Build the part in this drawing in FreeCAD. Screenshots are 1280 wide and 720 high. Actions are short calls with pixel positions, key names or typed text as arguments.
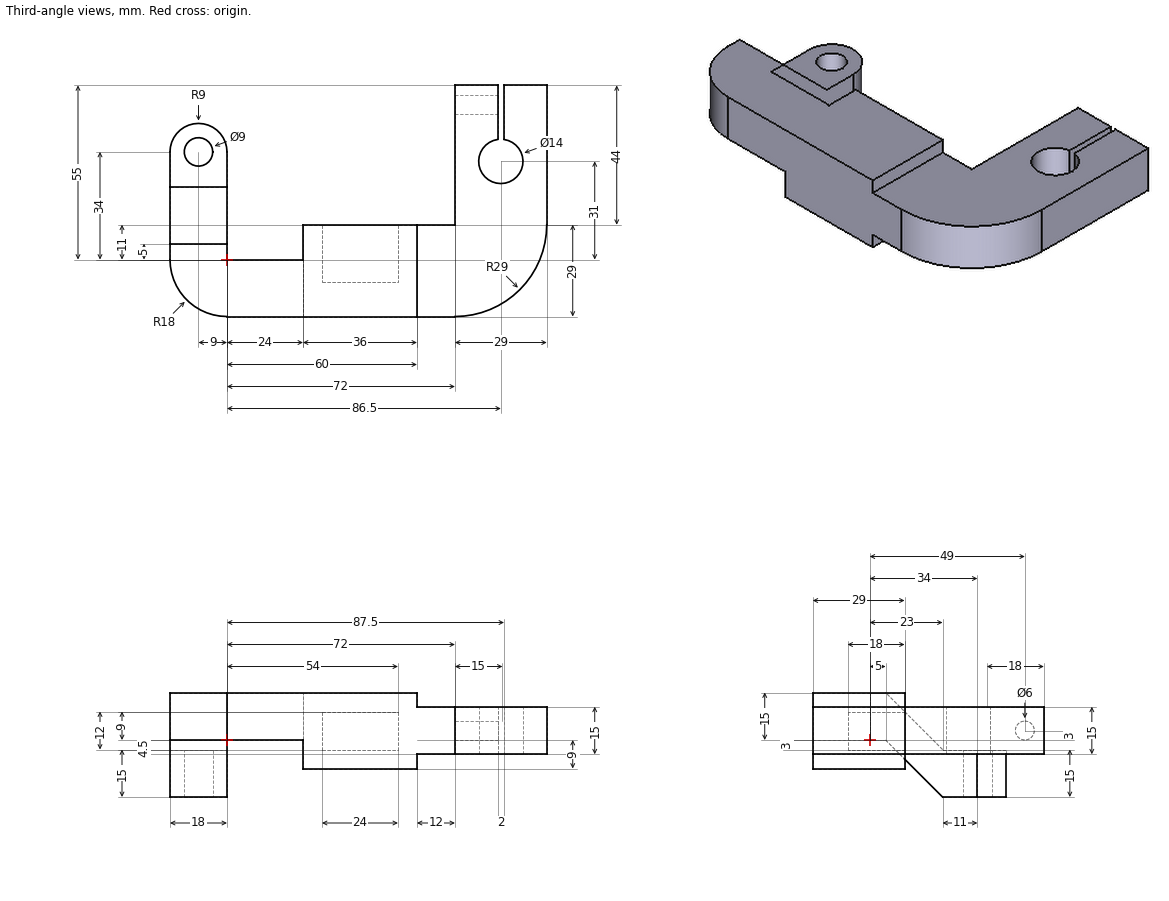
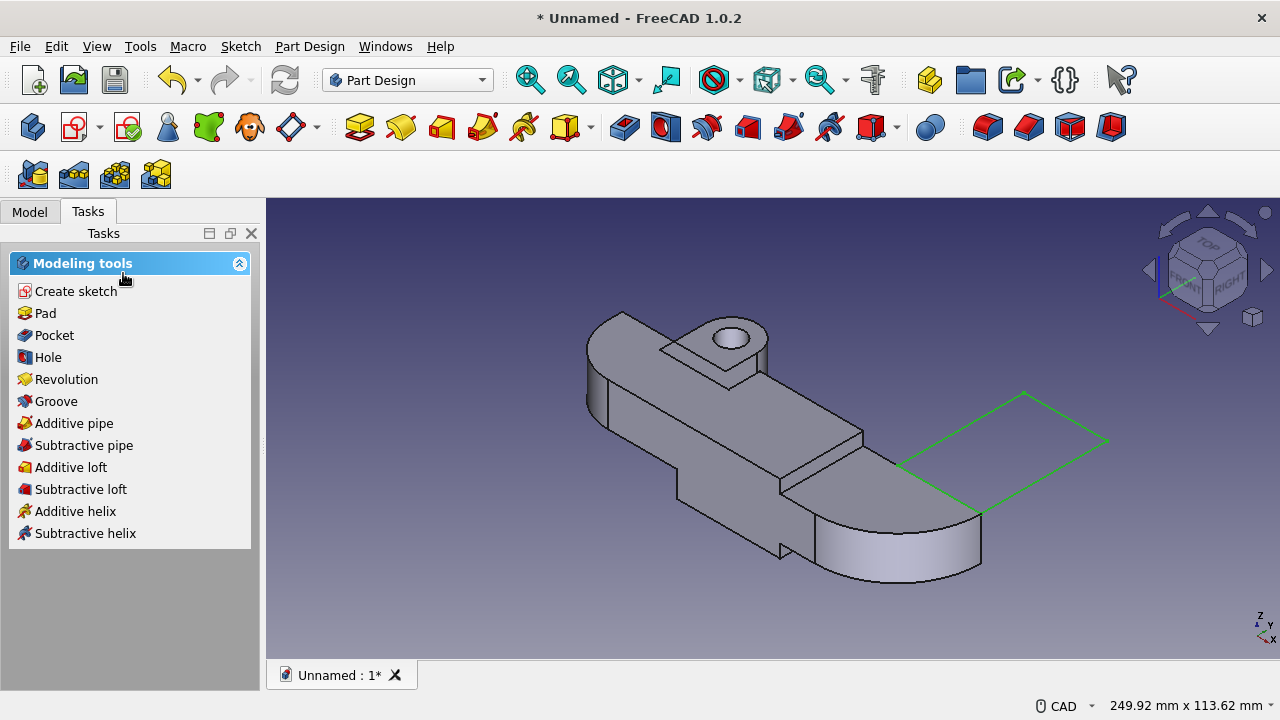
click(360, 128)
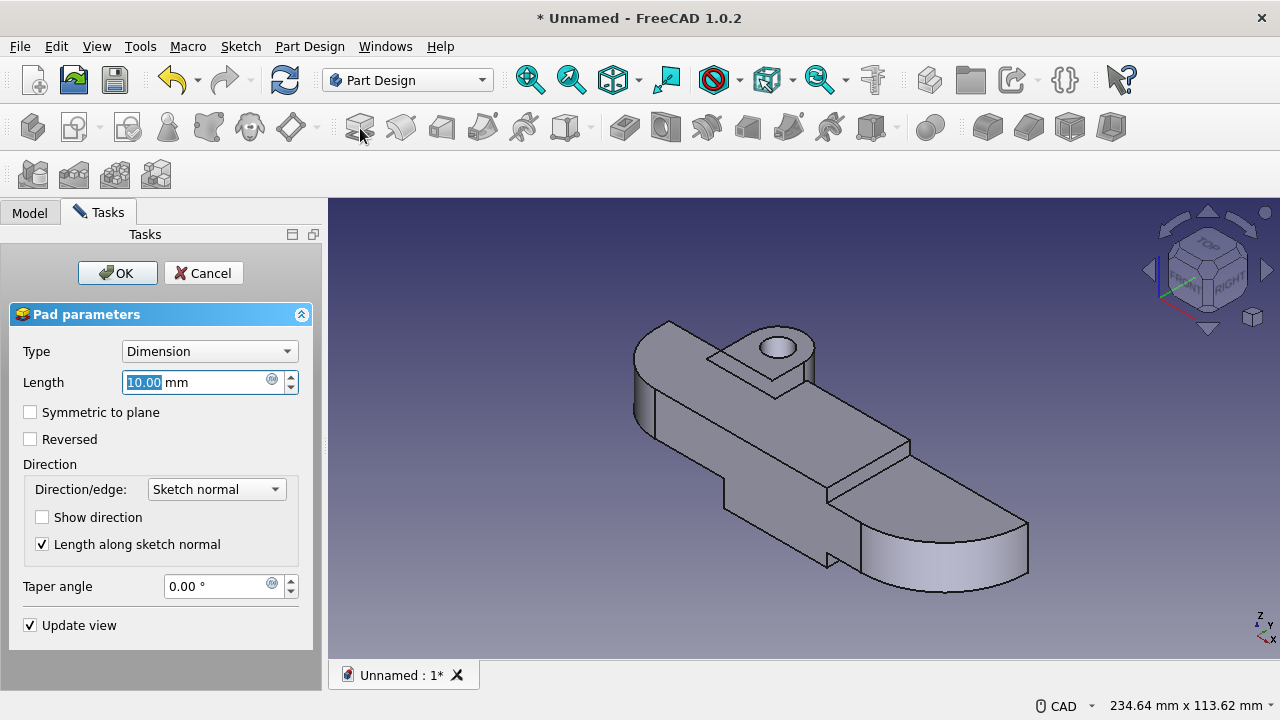
text(15)
key(Tab)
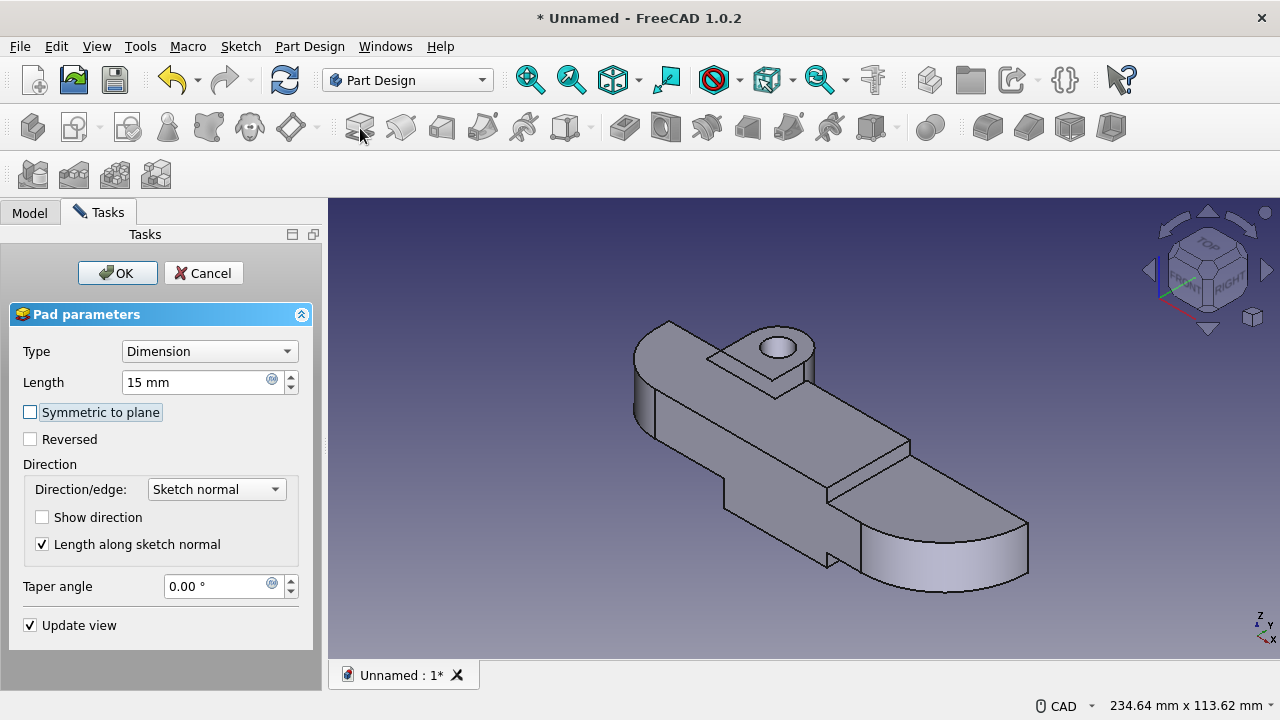
click(31, 439)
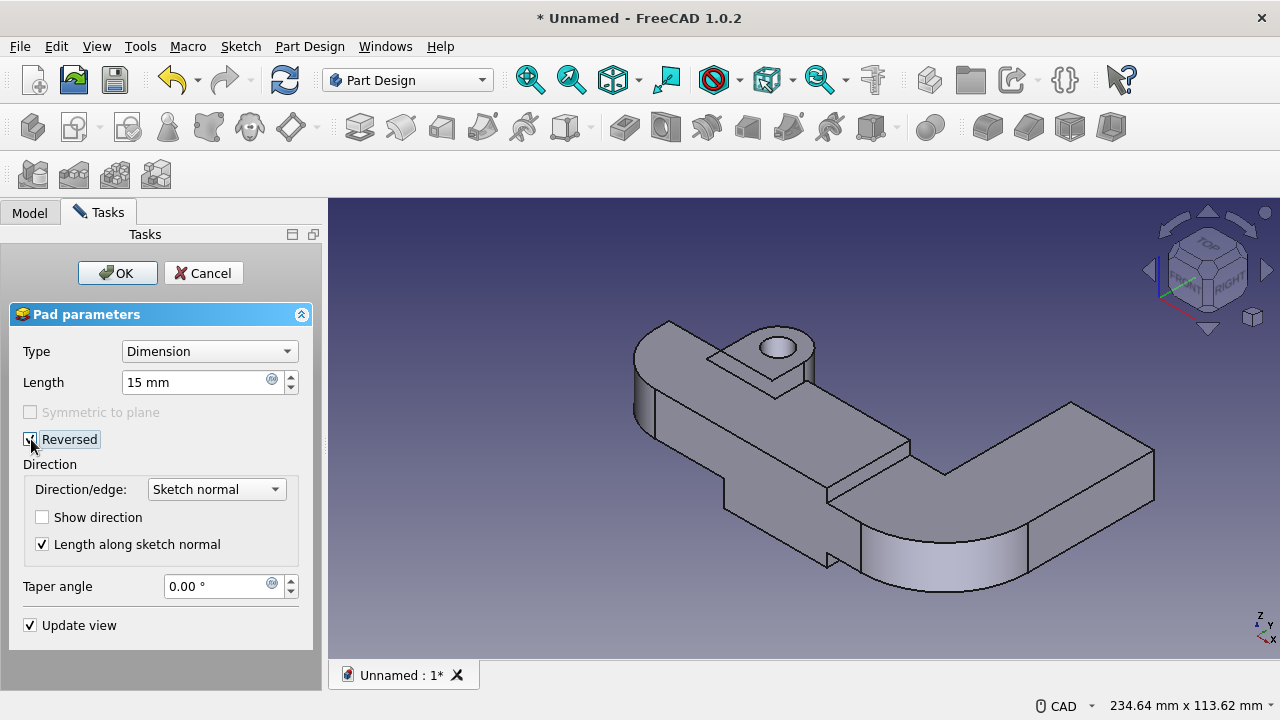
click(118, 273)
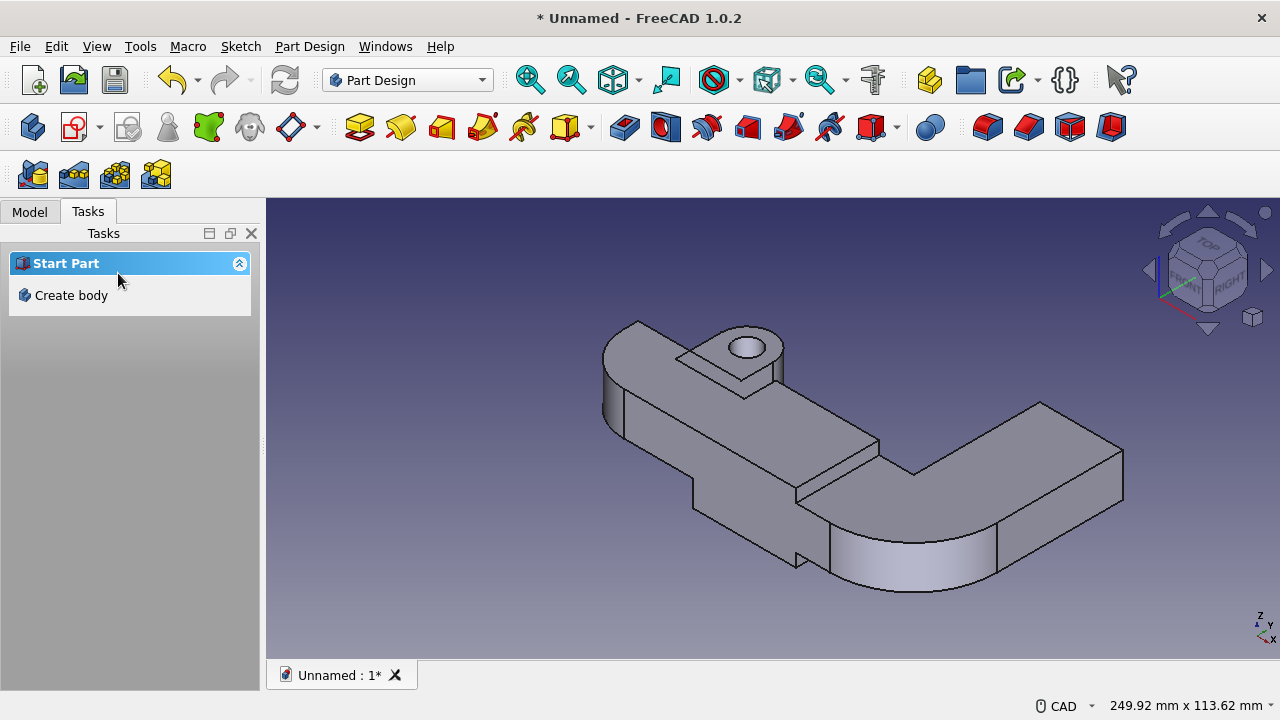
click(531, 80)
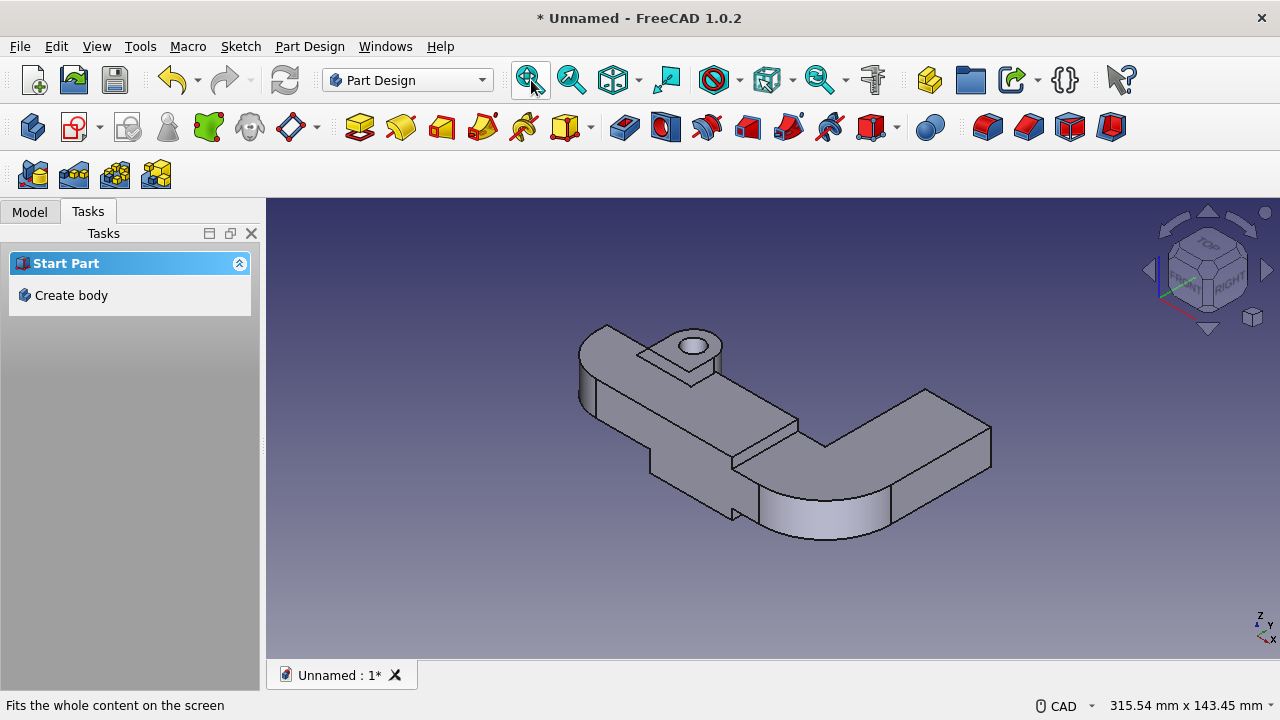
click(922, 427)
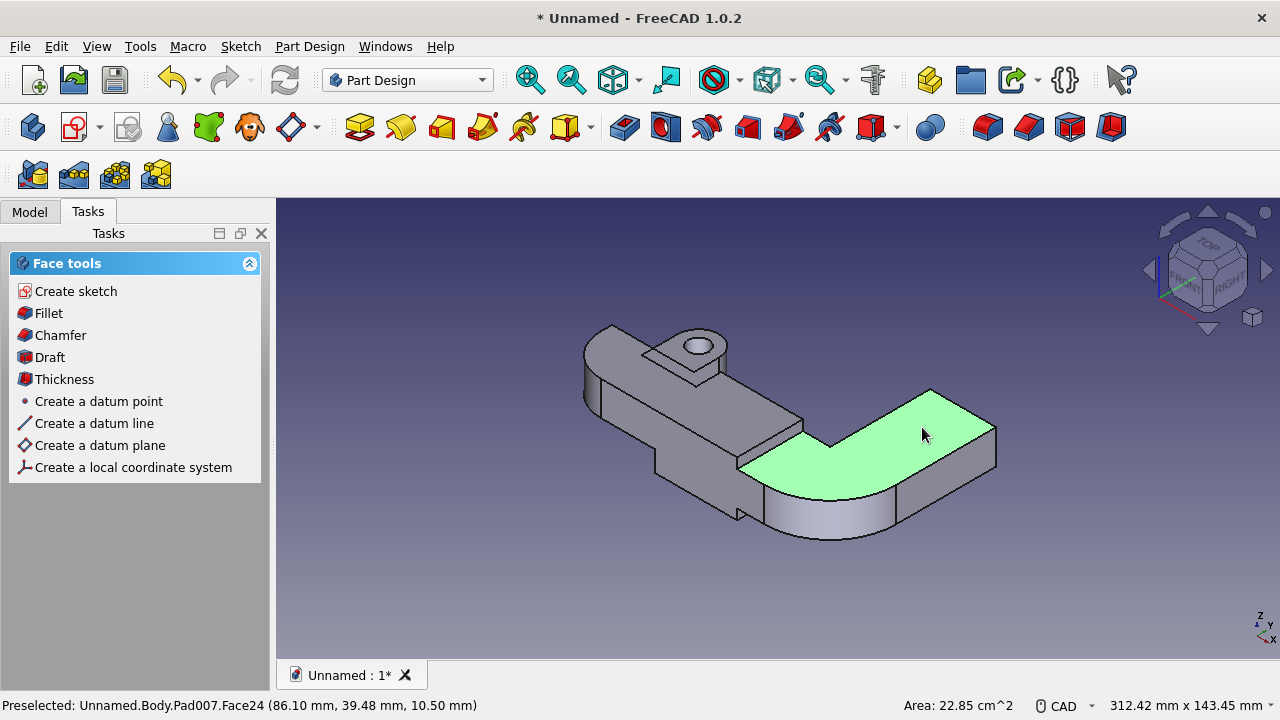
click(74, 128)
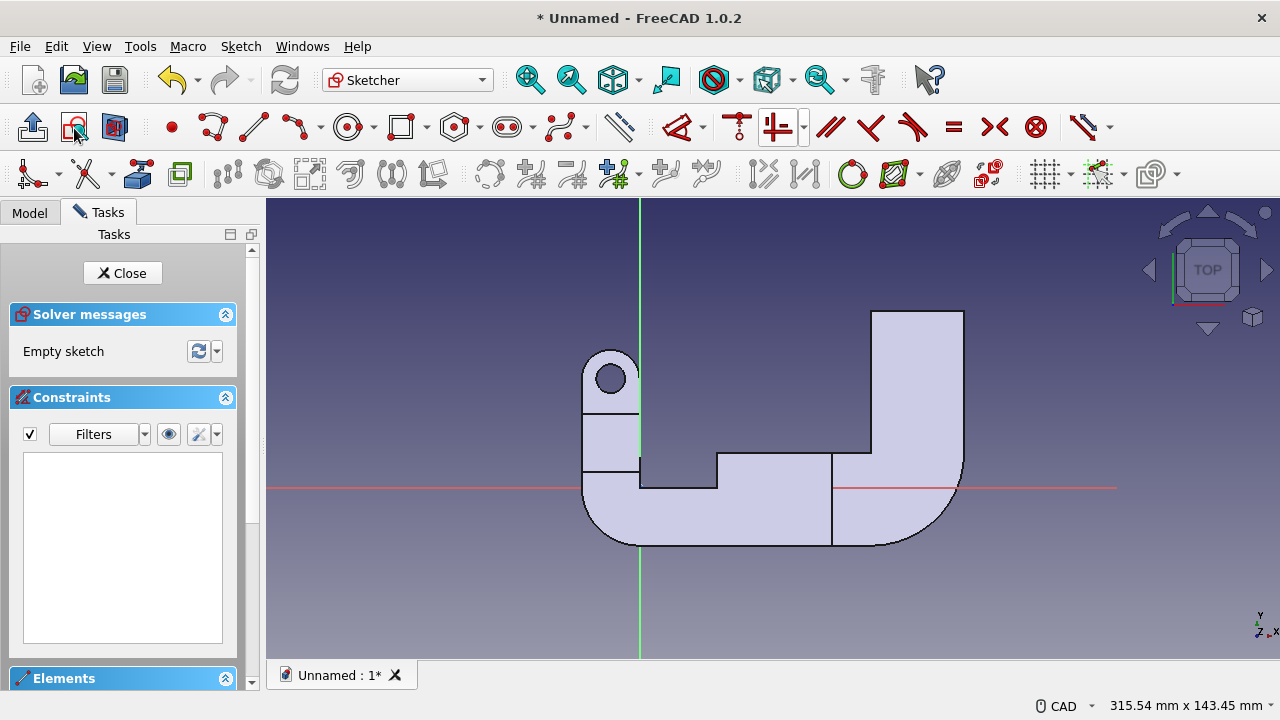
scroll(960, 380, up, 9)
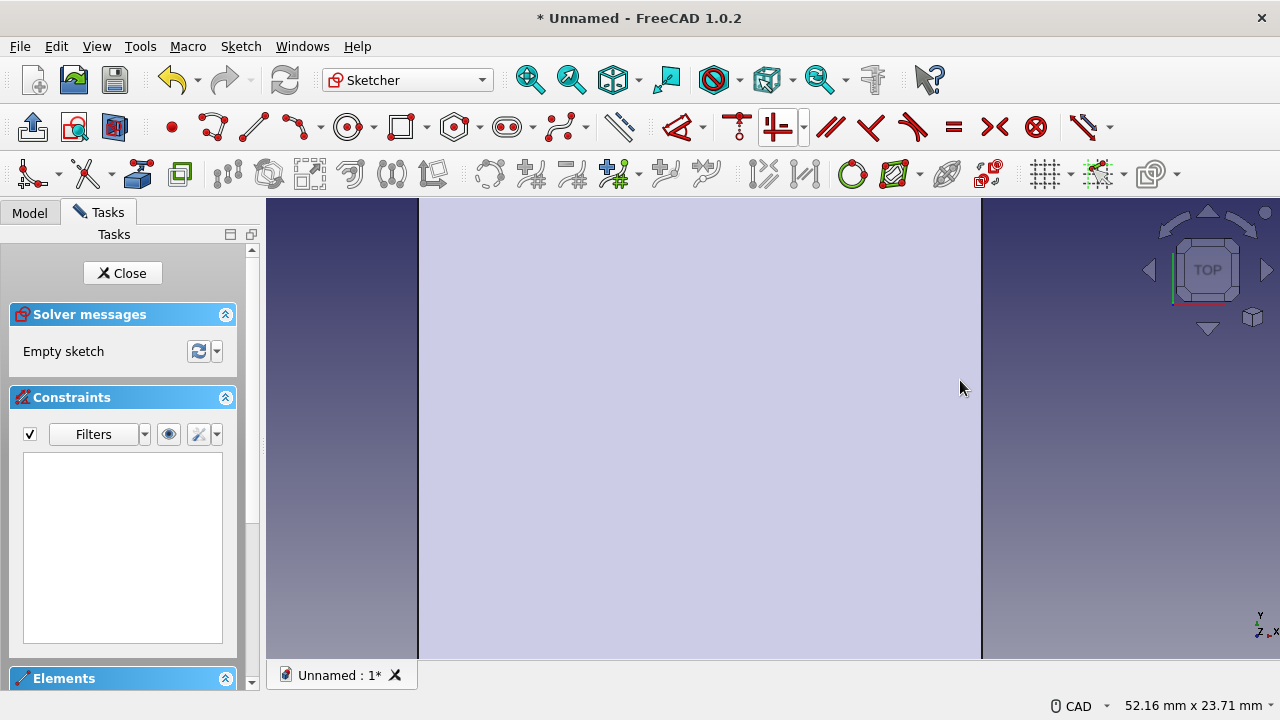
click(348, 128)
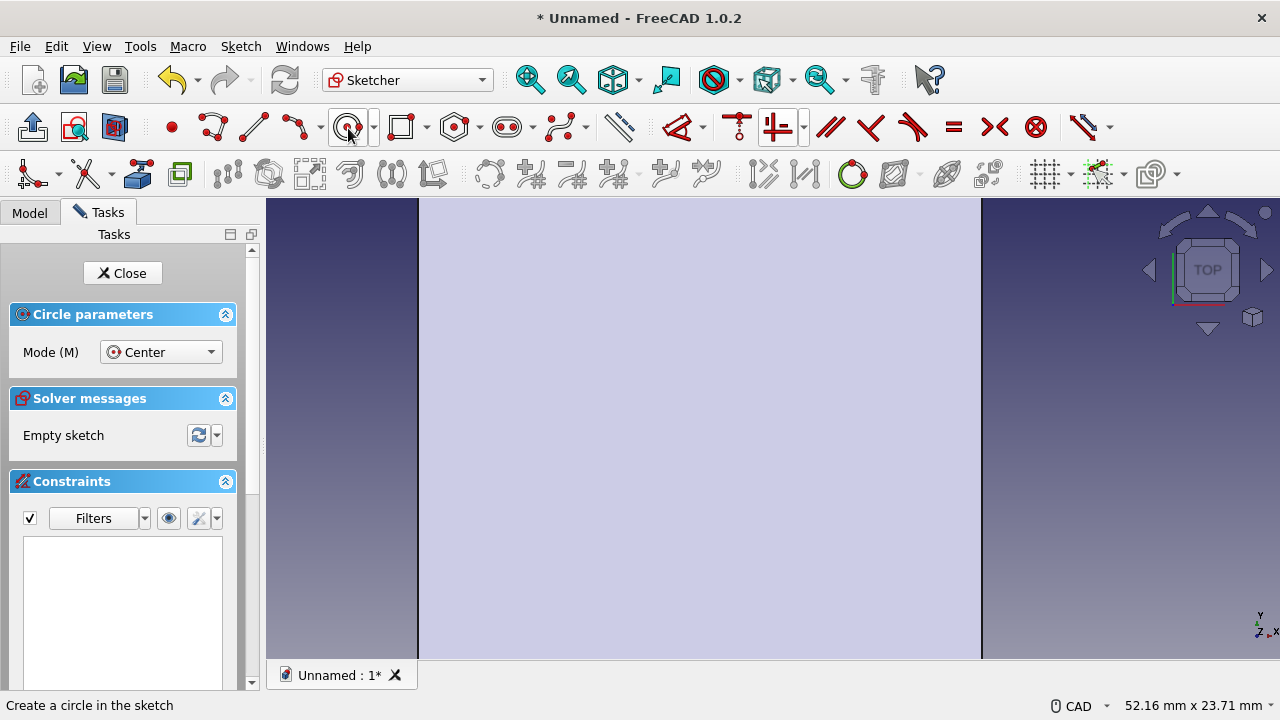
click(700, 428)
move(796, 332)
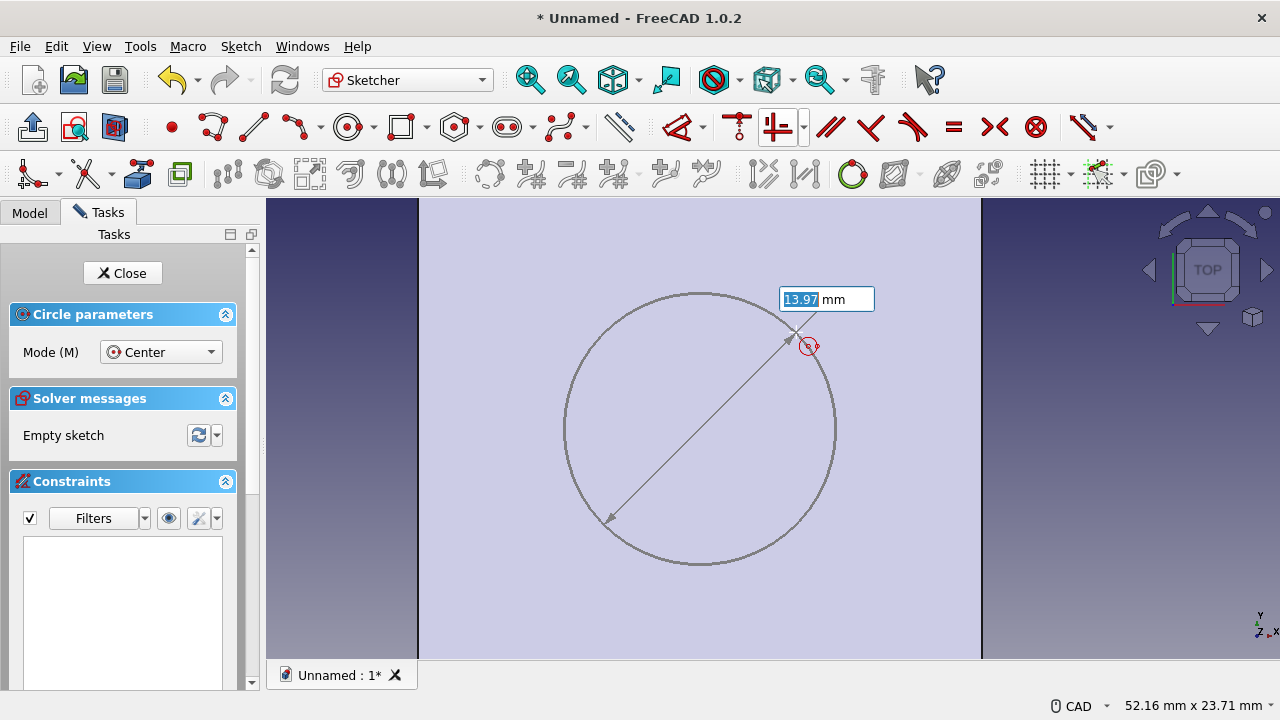
text(14)
key(Return)
key(Escape)